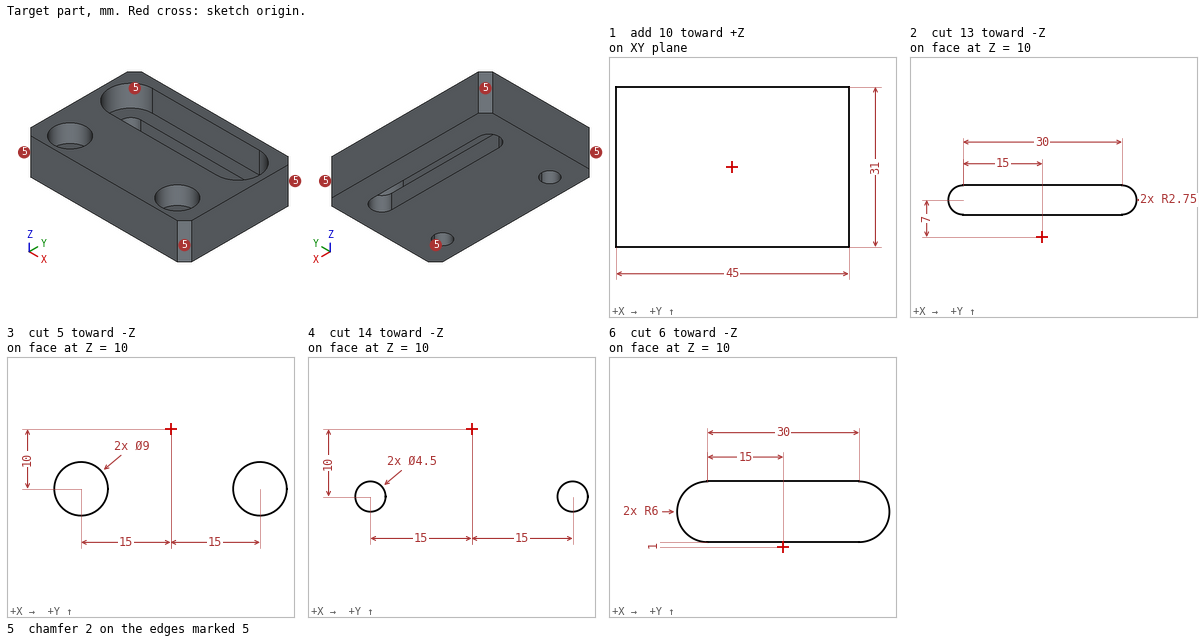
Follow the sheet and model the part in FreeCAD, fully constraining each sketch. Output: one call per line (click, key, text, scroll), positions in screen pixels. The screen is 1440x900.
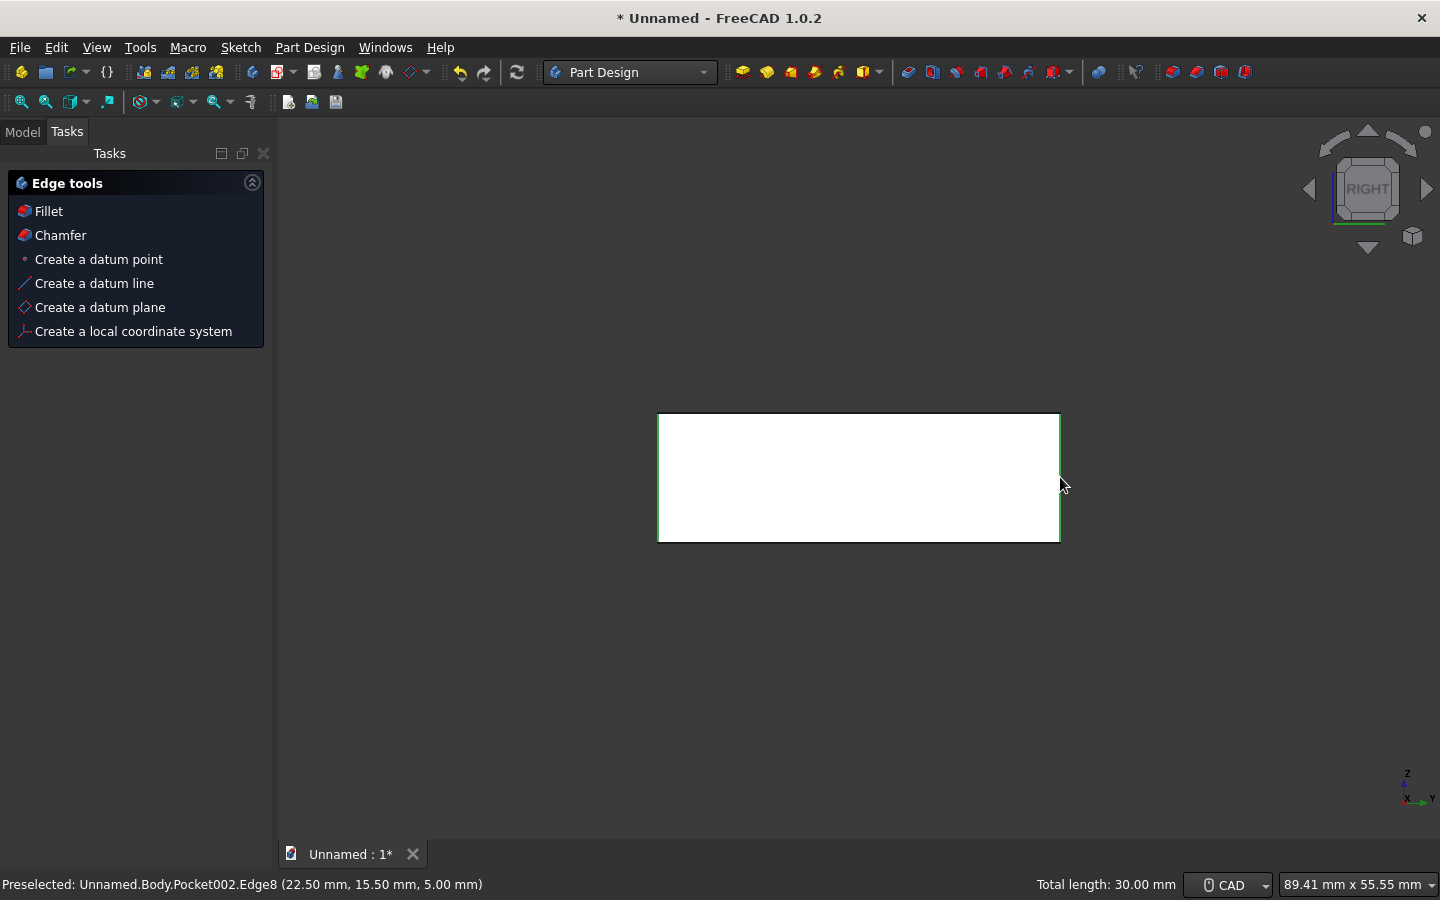
key(5)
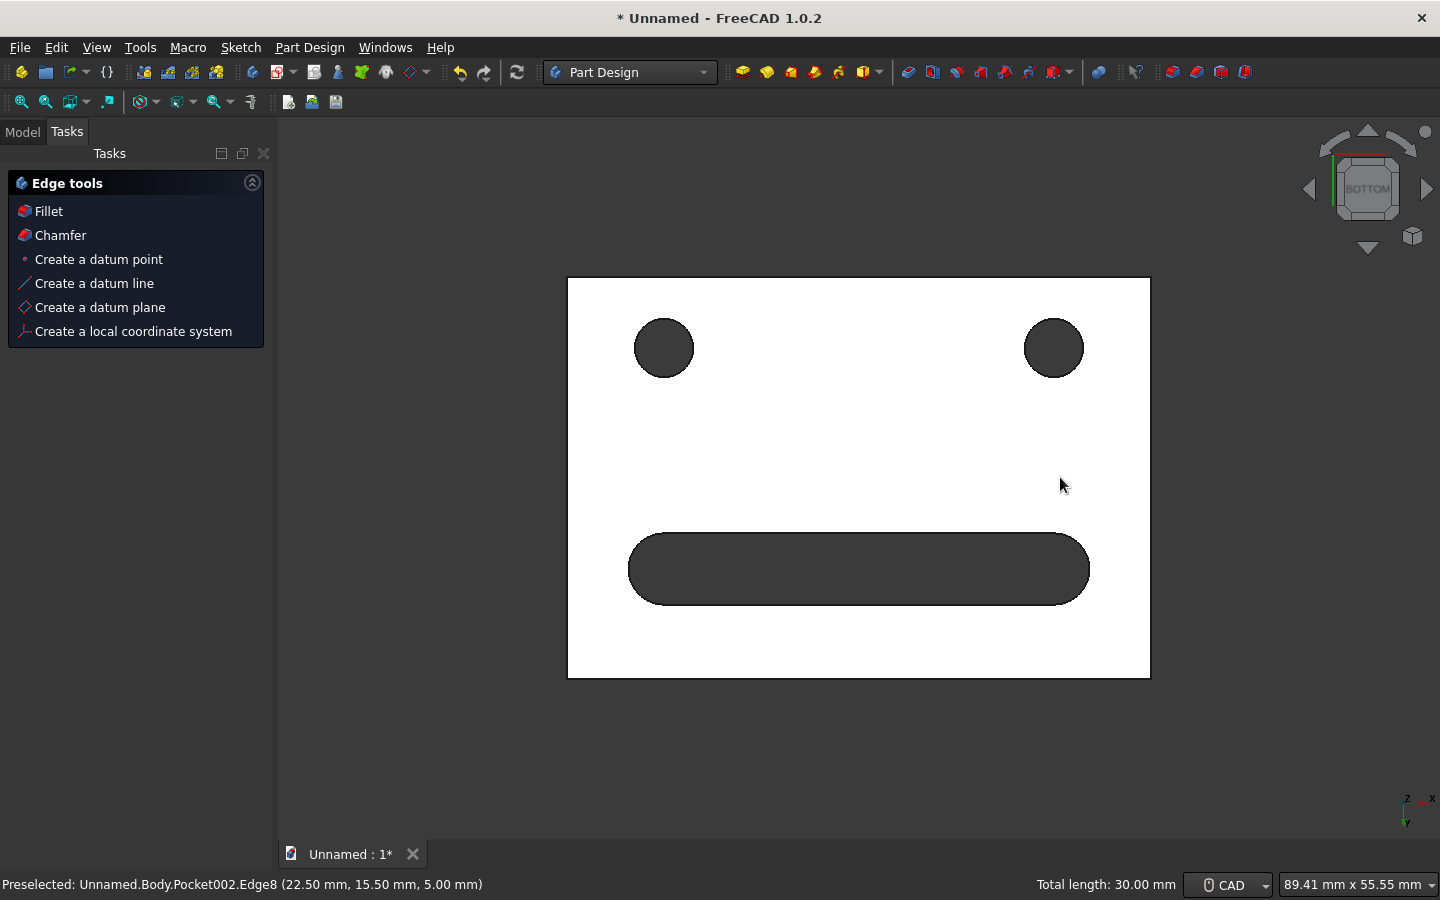
key(4)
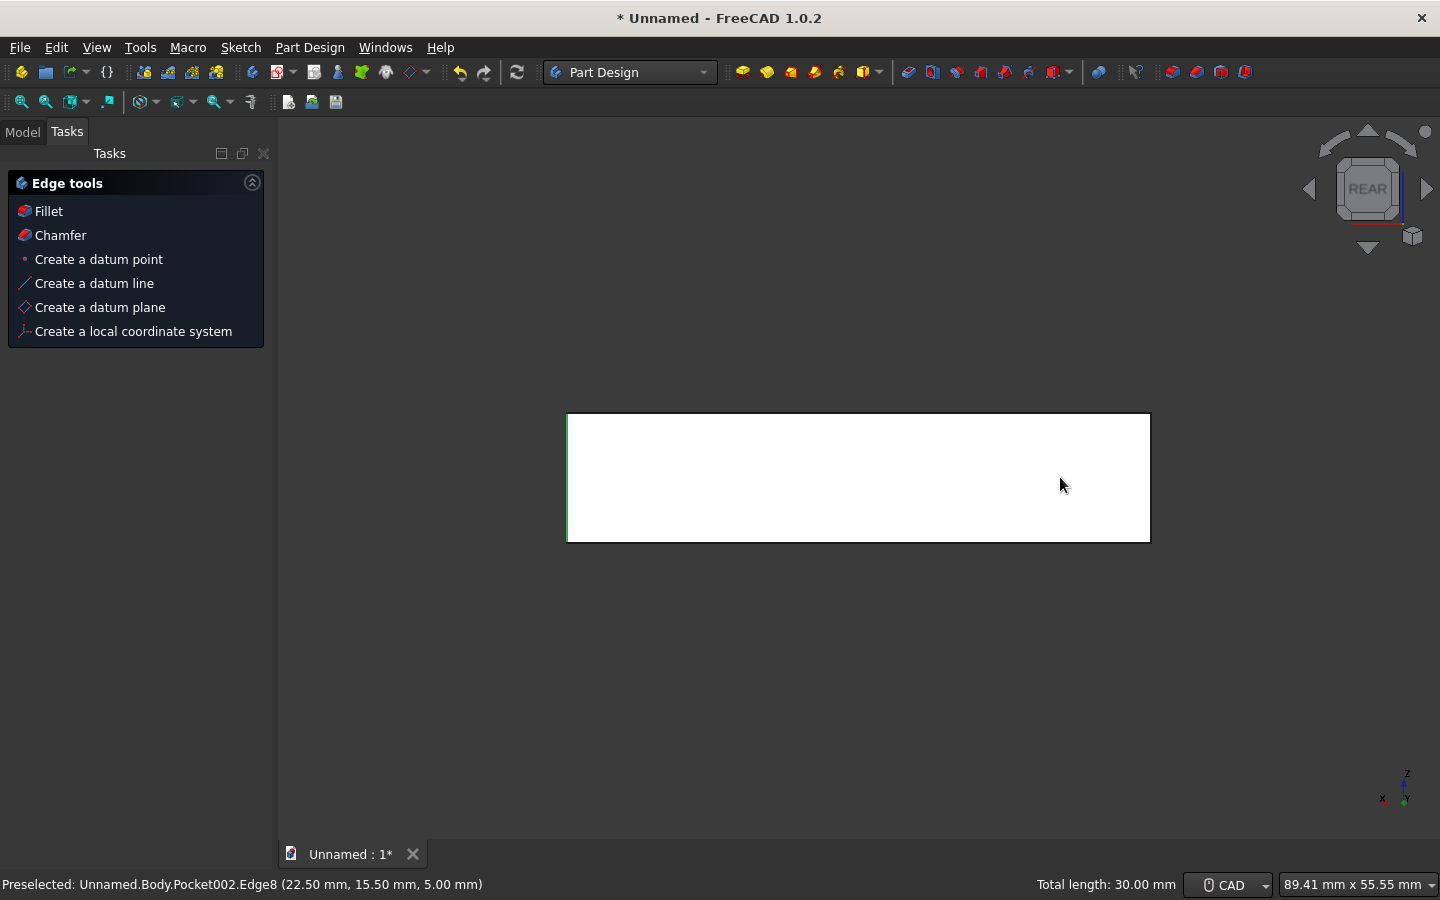
click(1151, 477, ctrl)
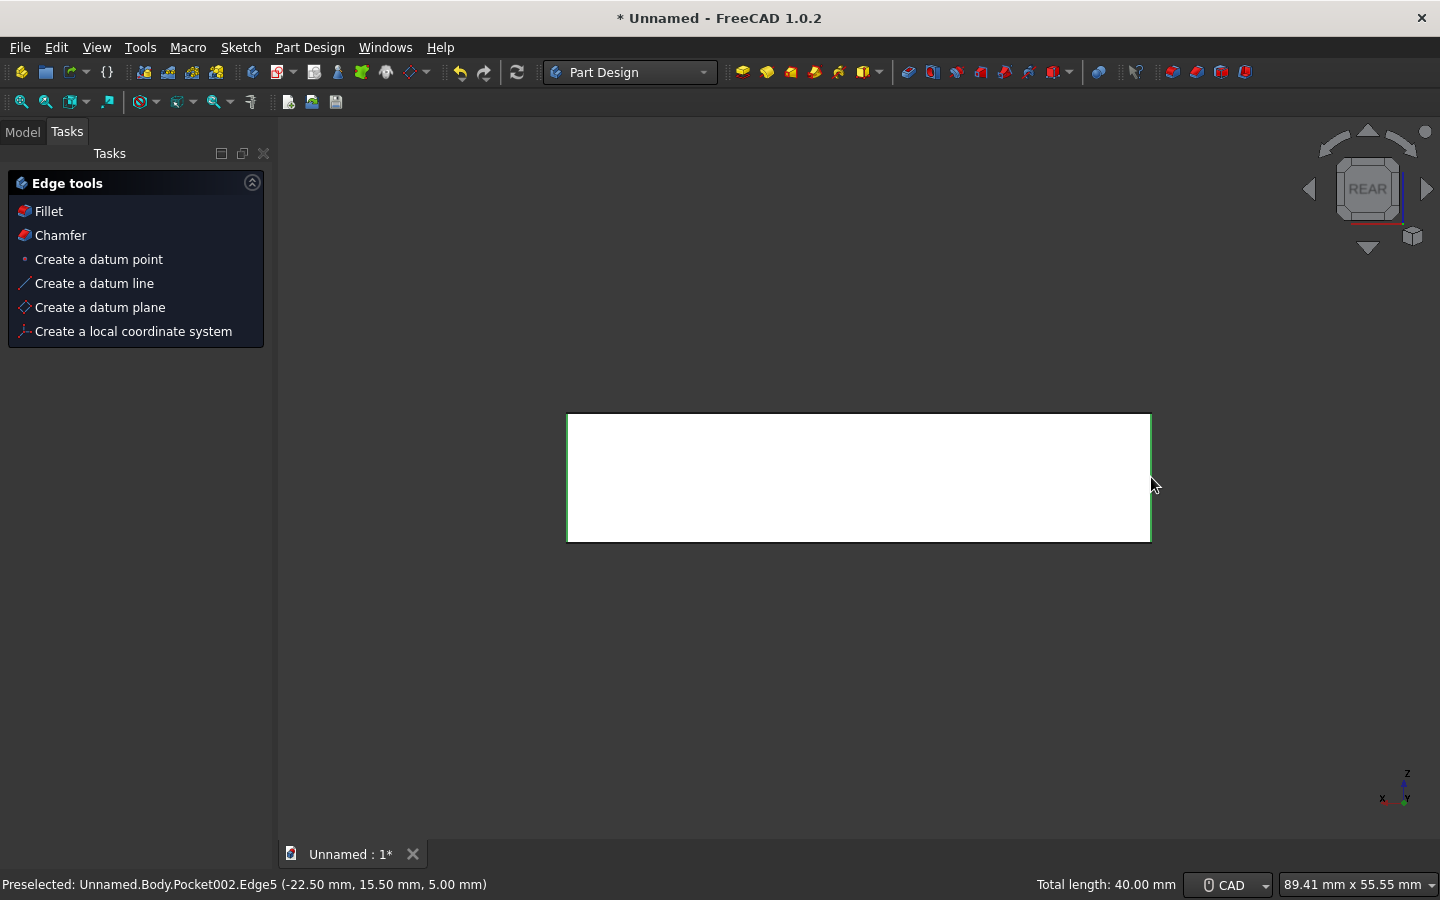
click(1198, 72)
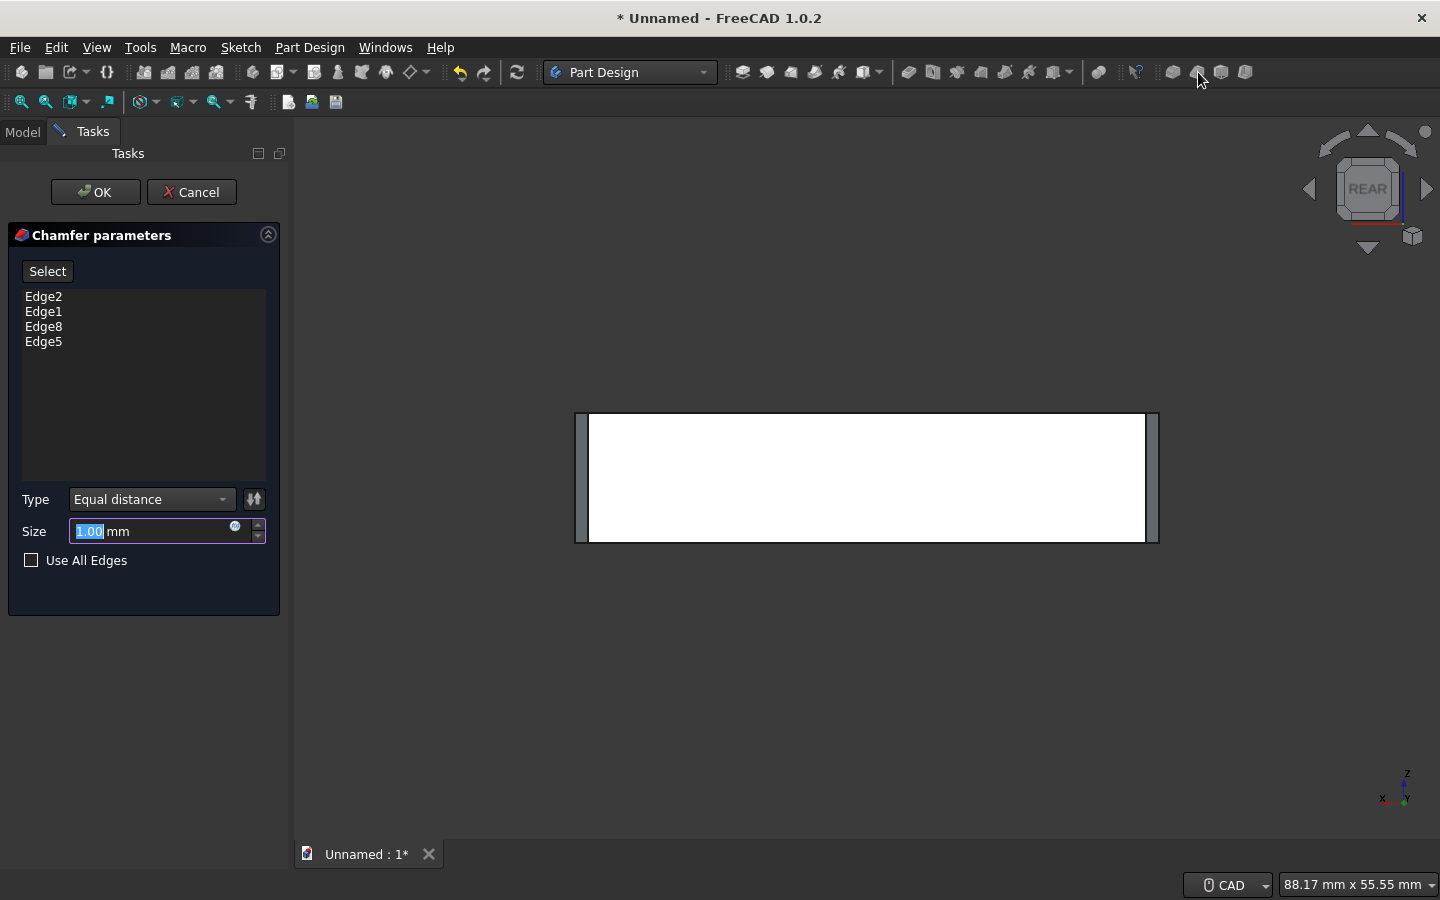
text(2)
key(Tab)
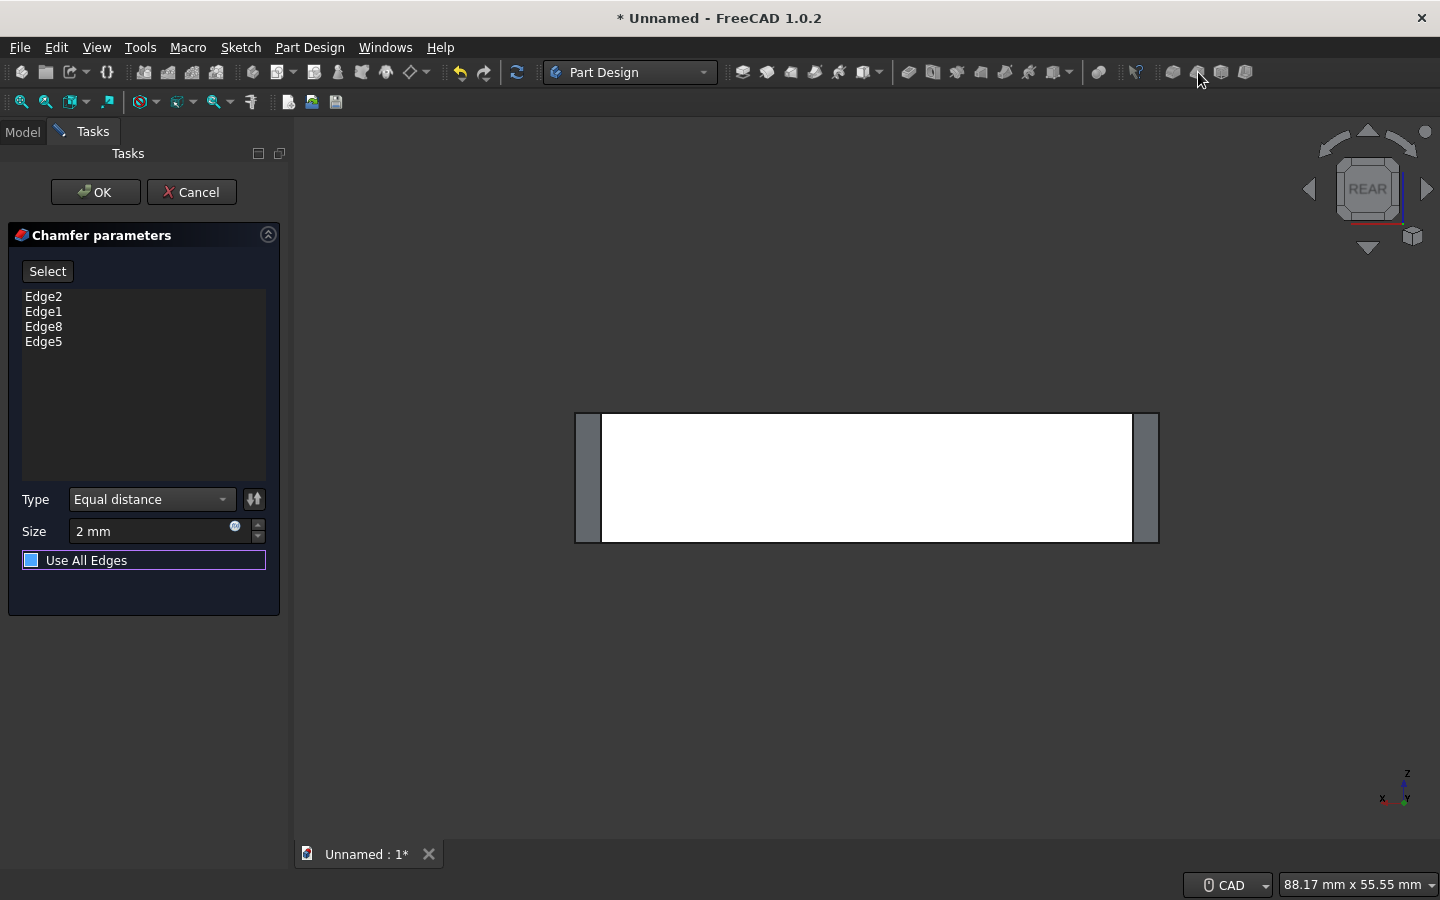
click(96, 192)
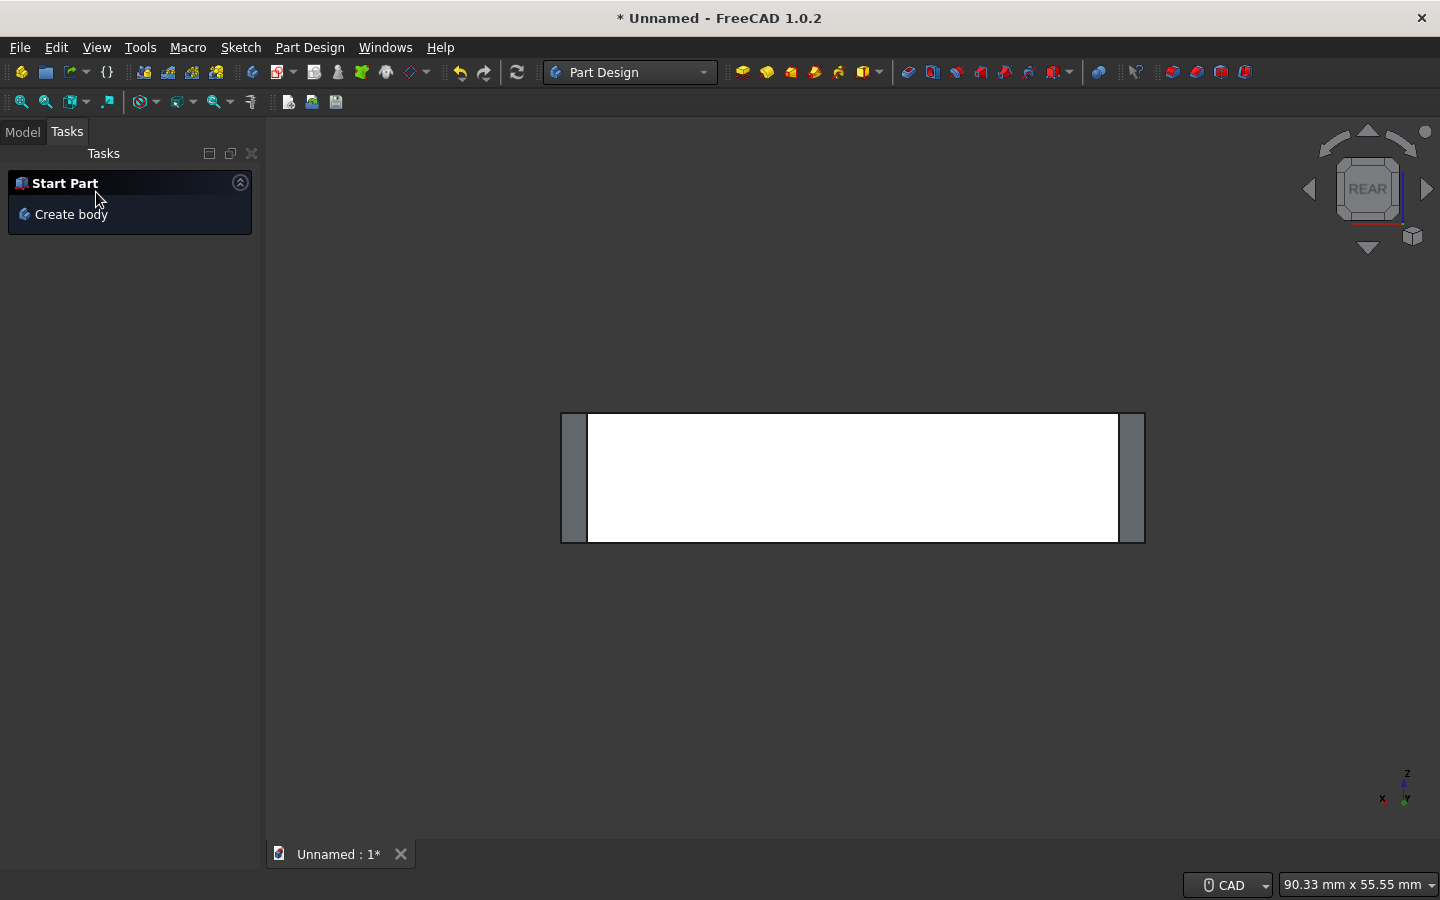
key(0)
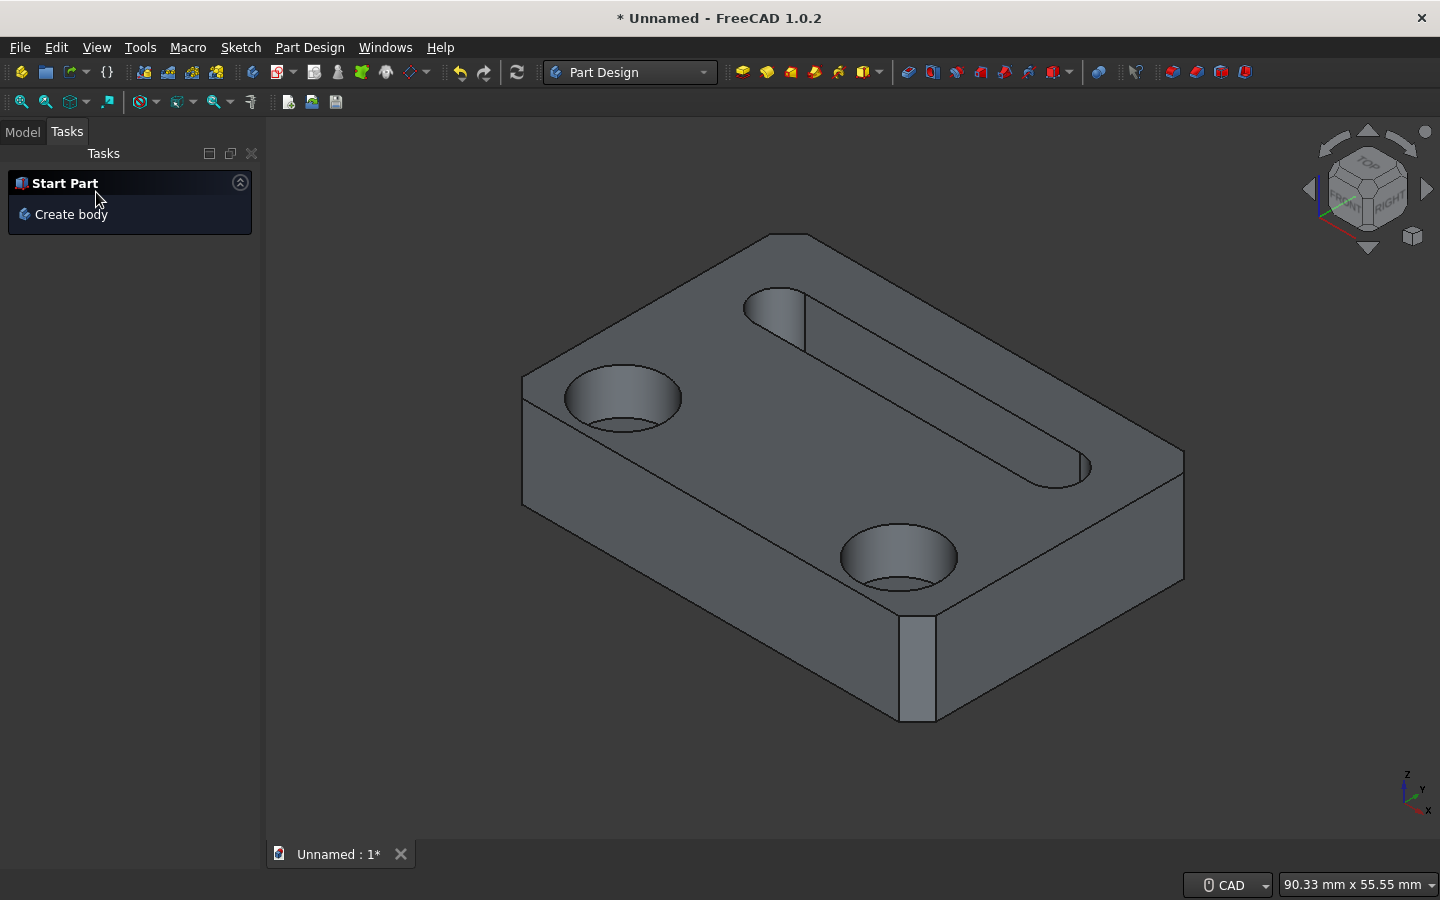
click(812, 447)